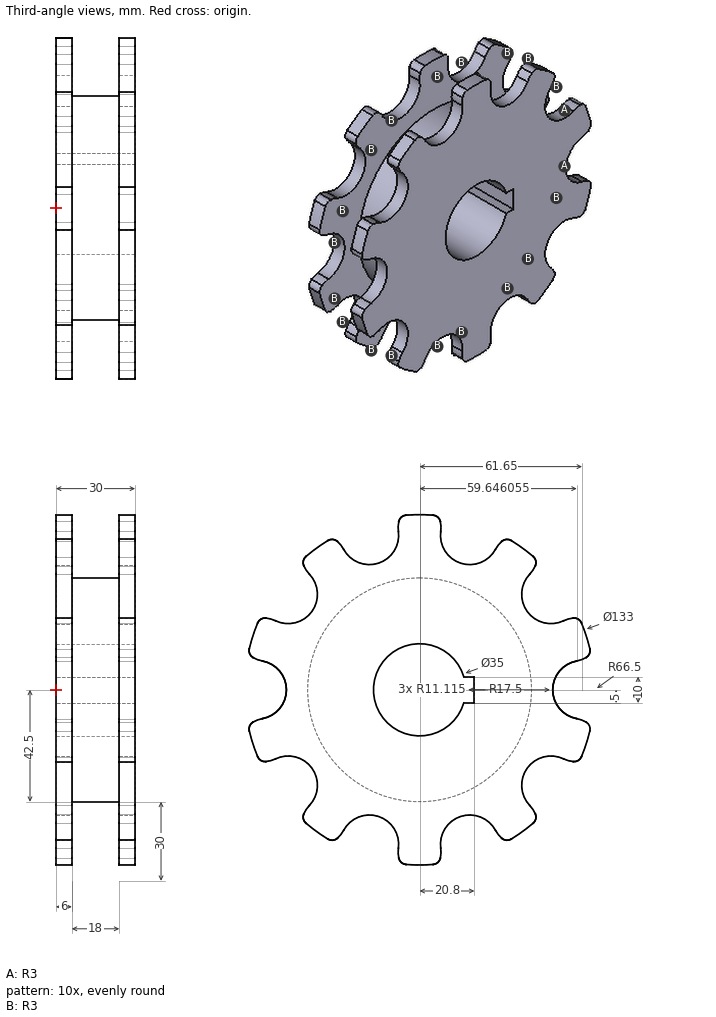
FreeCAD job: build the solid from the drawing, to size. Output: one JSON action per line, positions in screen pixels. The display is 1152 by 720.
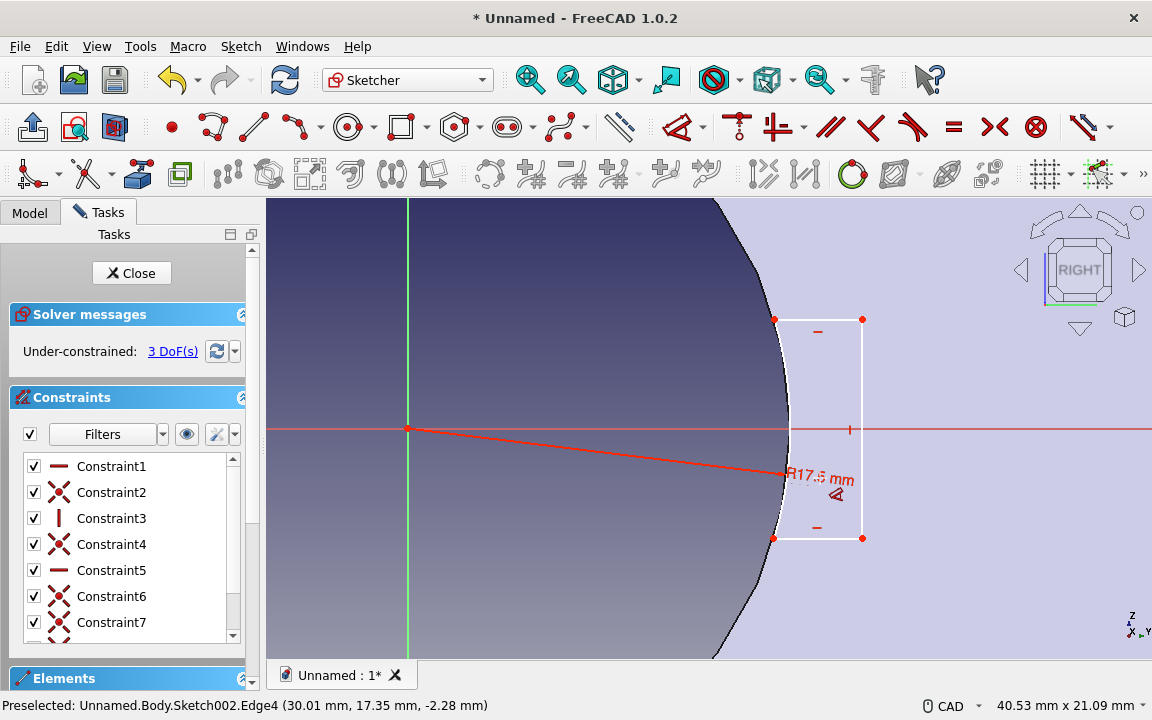
{"action": "left_click", "coordinate": [862, 473]}
{"action": "left_click", "coordinate": [896, 379]}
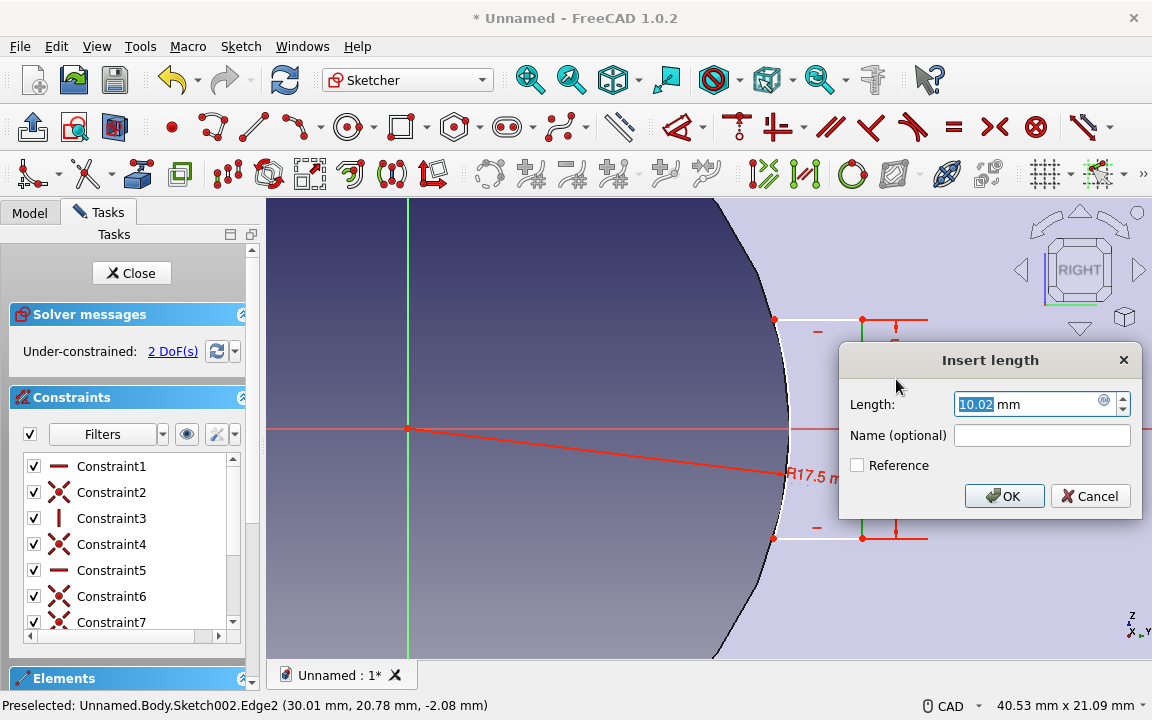
{"action": "type", "text": "10"}
{"action": "key", "text": "Return"}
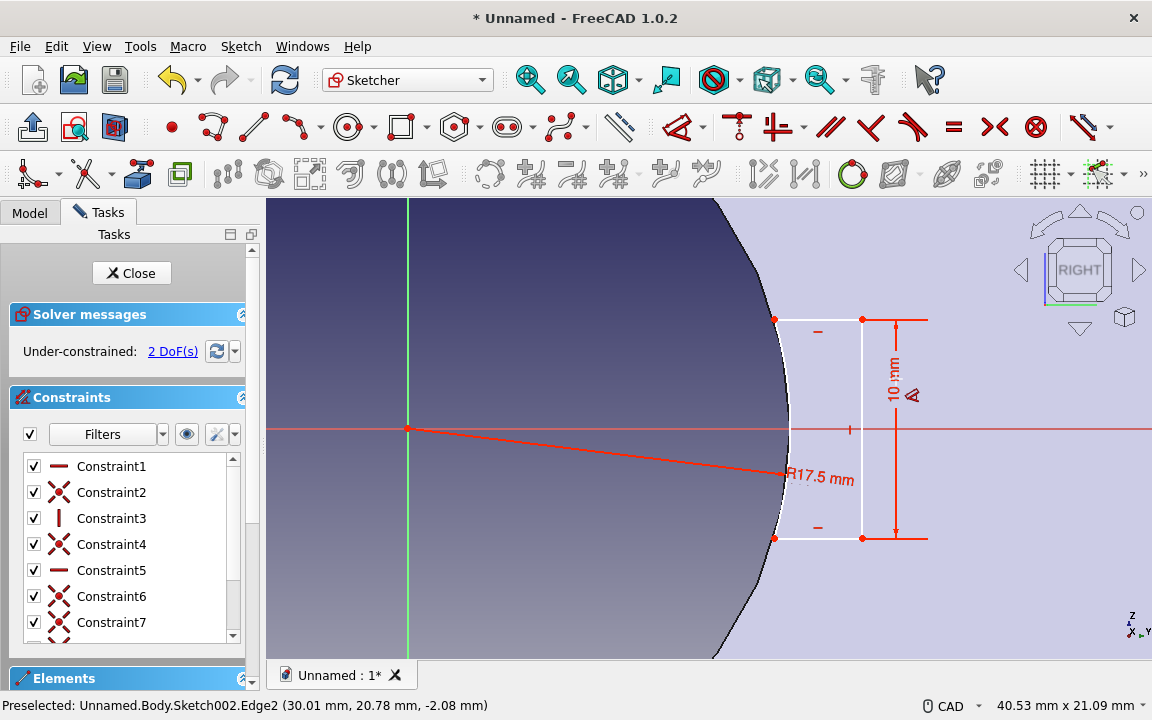
{"action": "left_click", "coordinate": [774, 539]}
{"action": "left_click", "coordinate": [374, 484]}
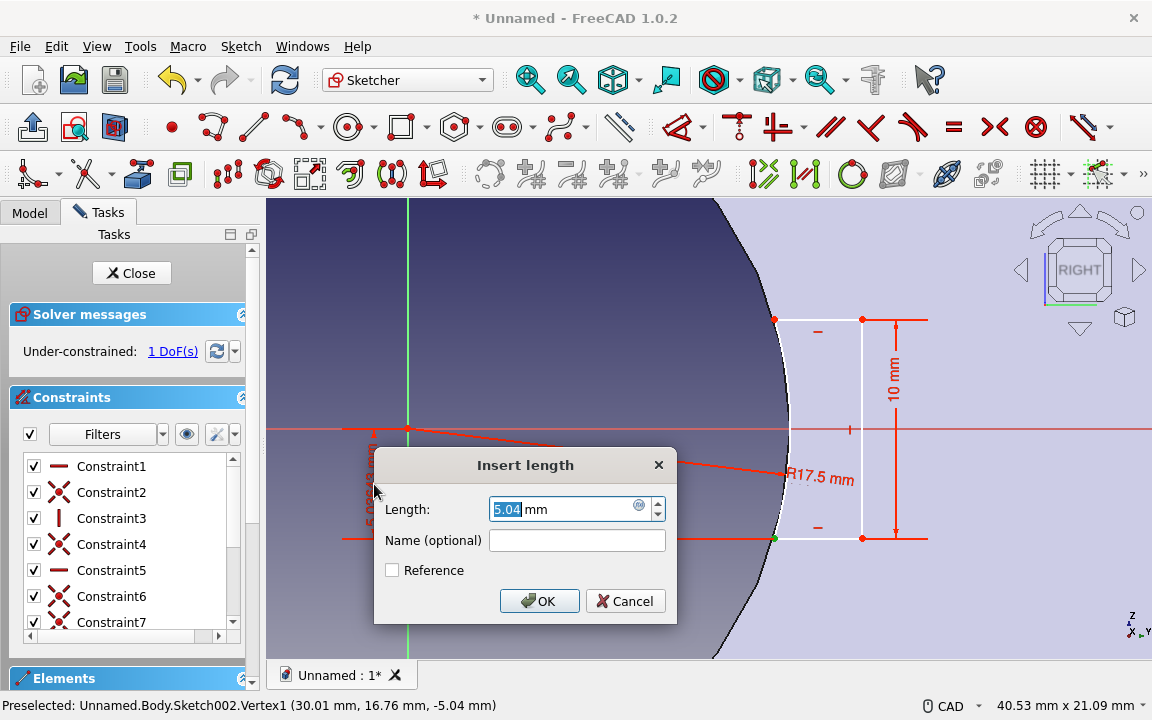
{"action": "type", "text": "5"}
{"action": "key", "text": "Return"}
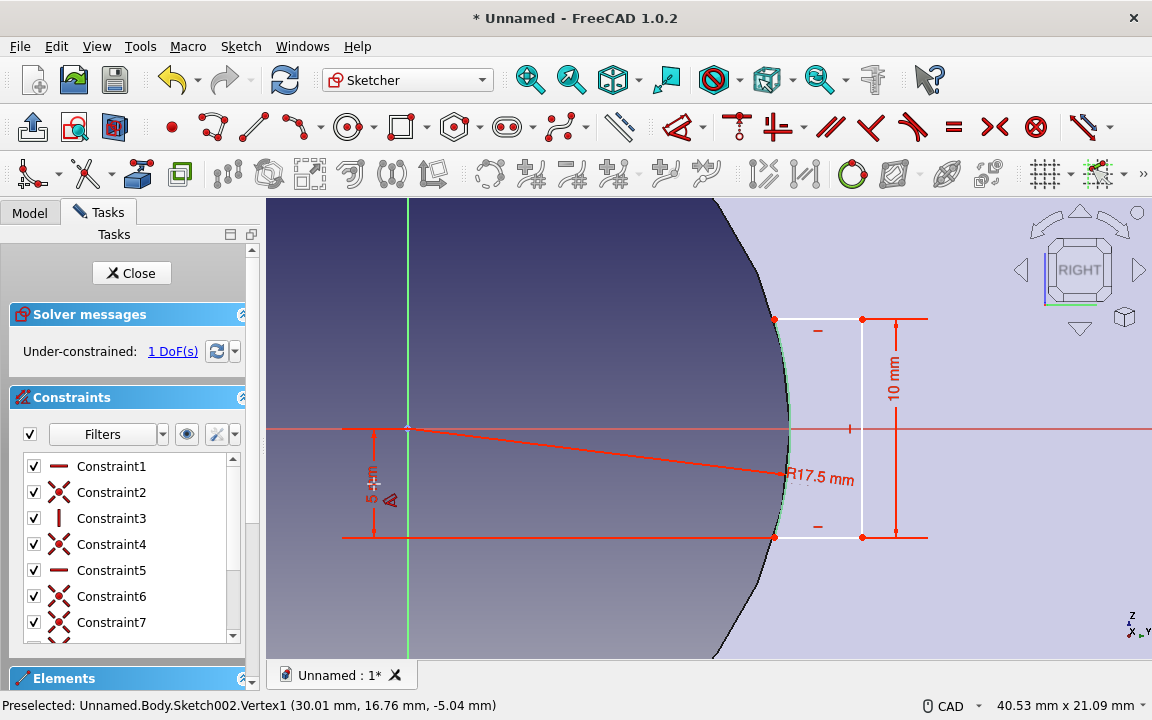
{"action": "left_click", "coordinate": [862, 538]}
{"action": "left_click", "coordinate": [635, 572]}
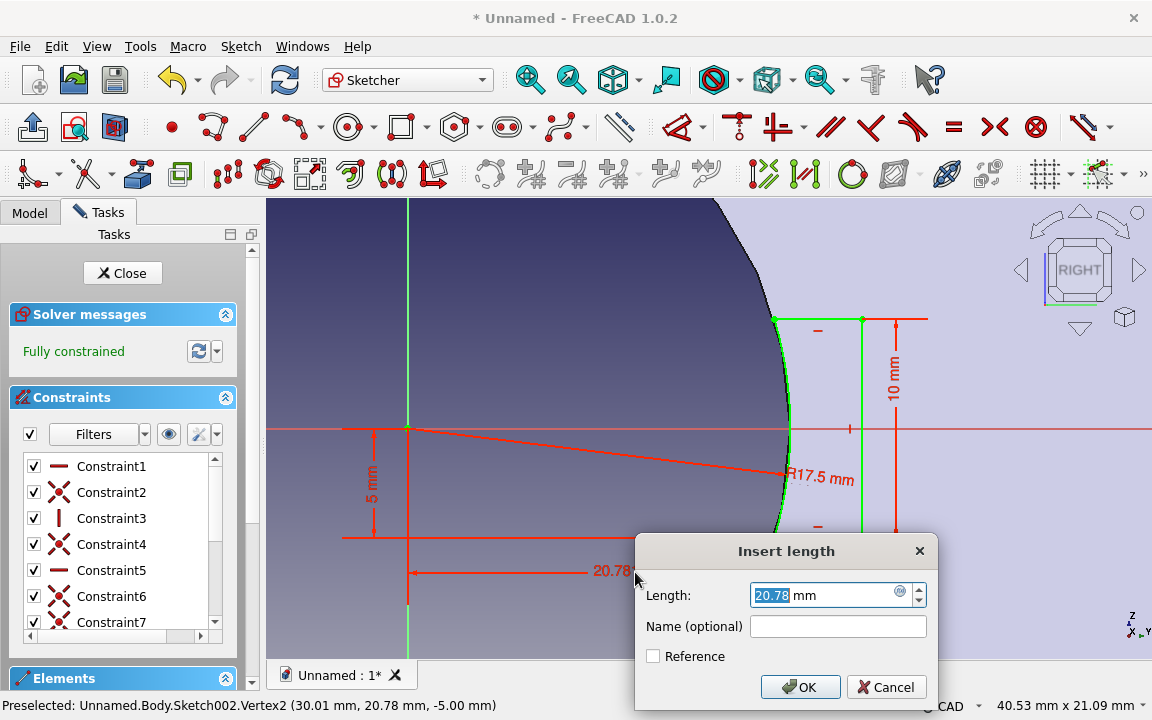
{"action": "type", "text": "20.8"}
{"action": "key", "text": "Return"}
{"action": "key", "text": "Escape"}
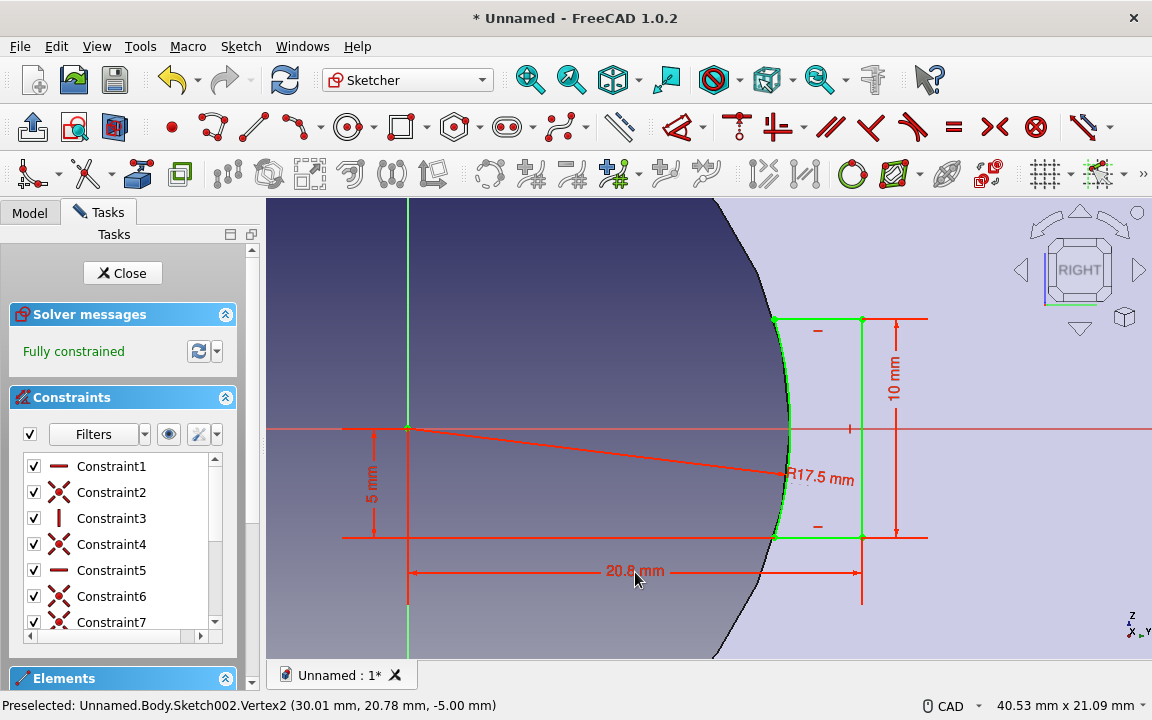
{"action": "left_click", "coordinate": [123, 273]}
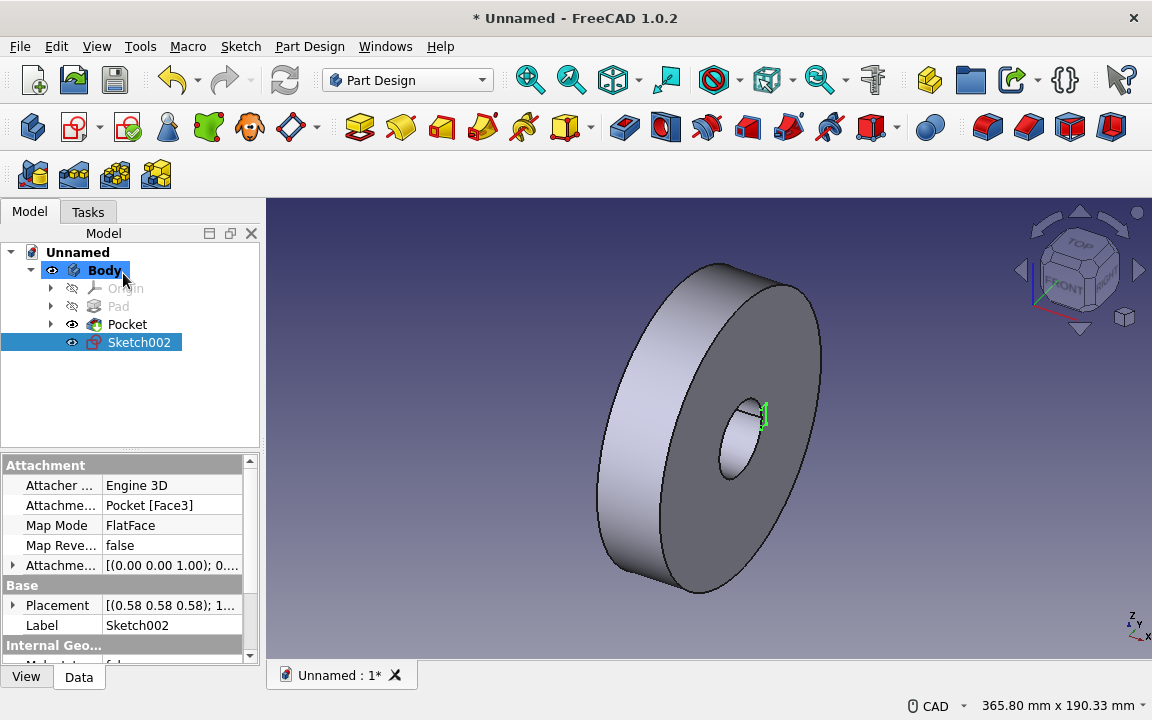
{"action": "left_click", "coordinate": [625, 128]}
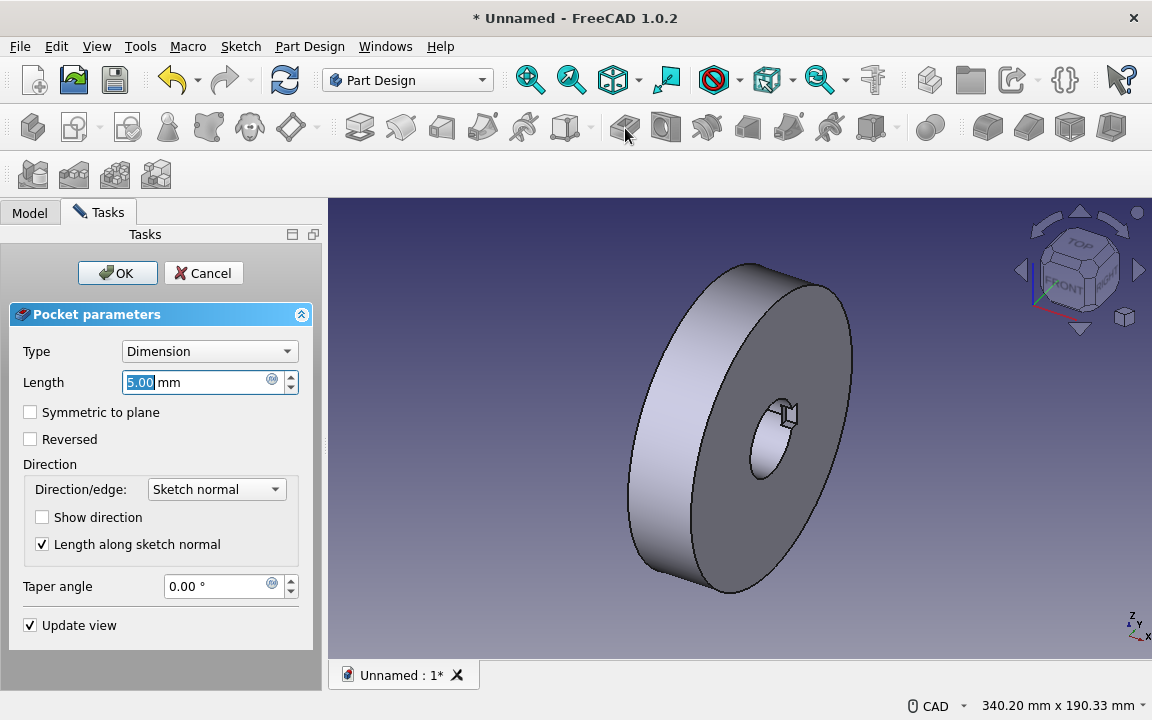
{"action": "left_click", "coordinate": [210, 352]}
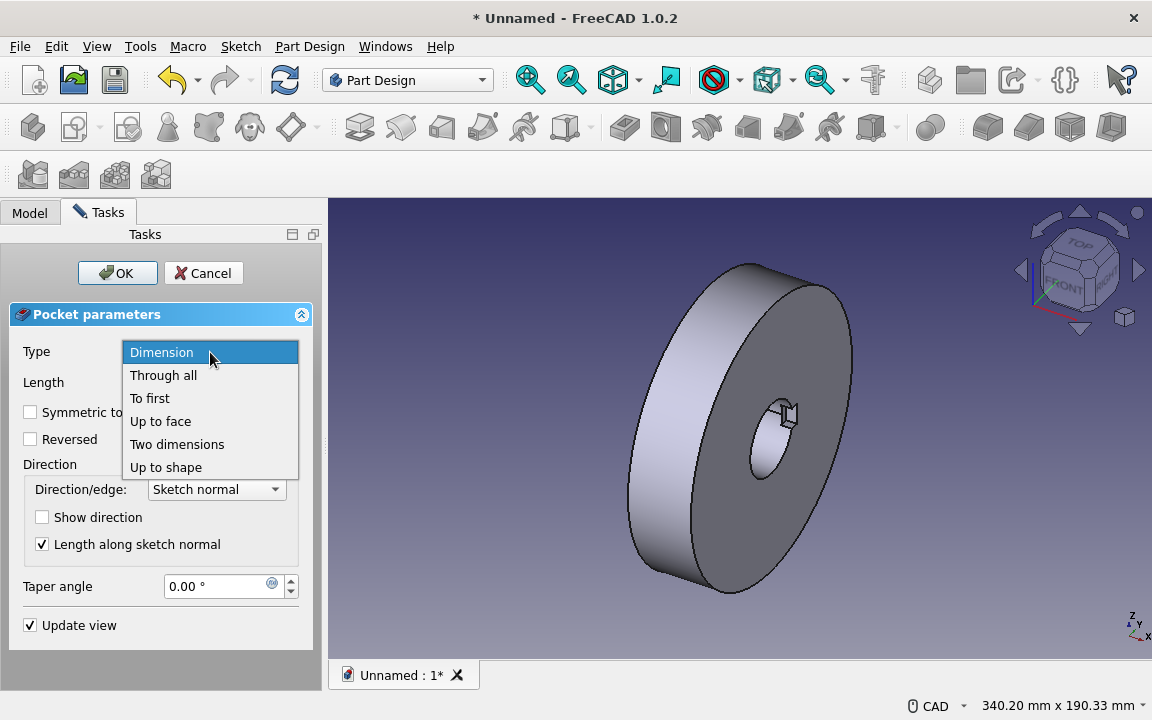
{"action": "left_click", "coordinate": [208, 376]}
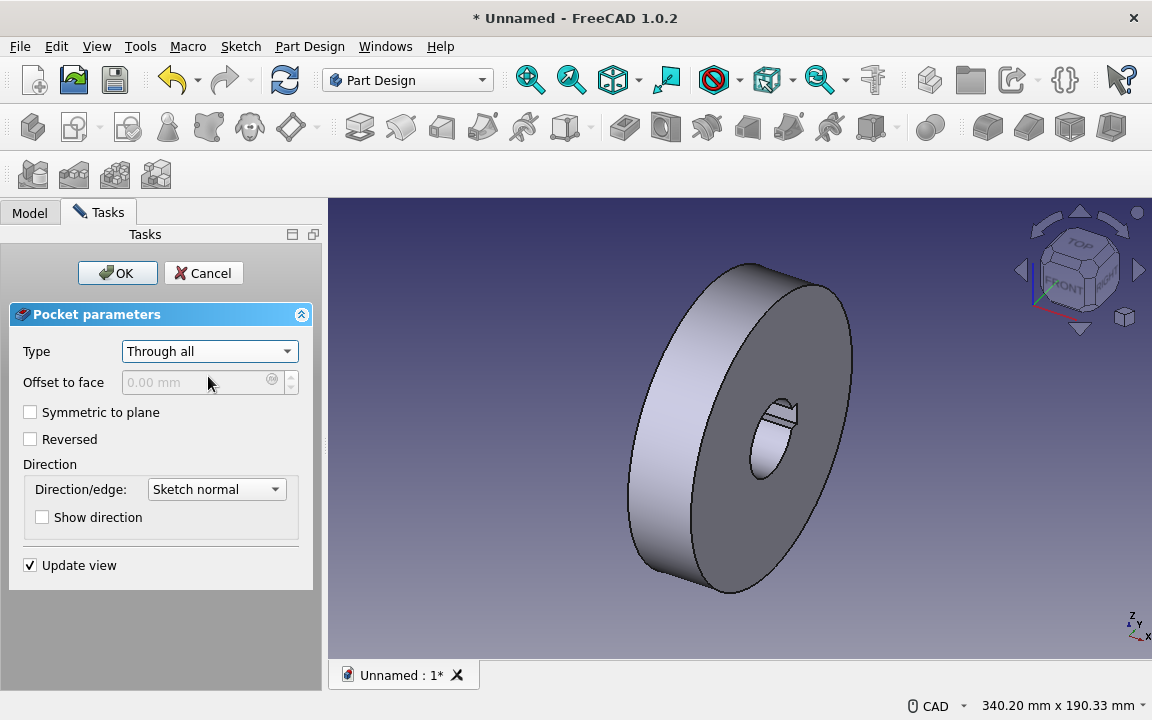
{"action": "left_click", "coordinate": [118, 273]}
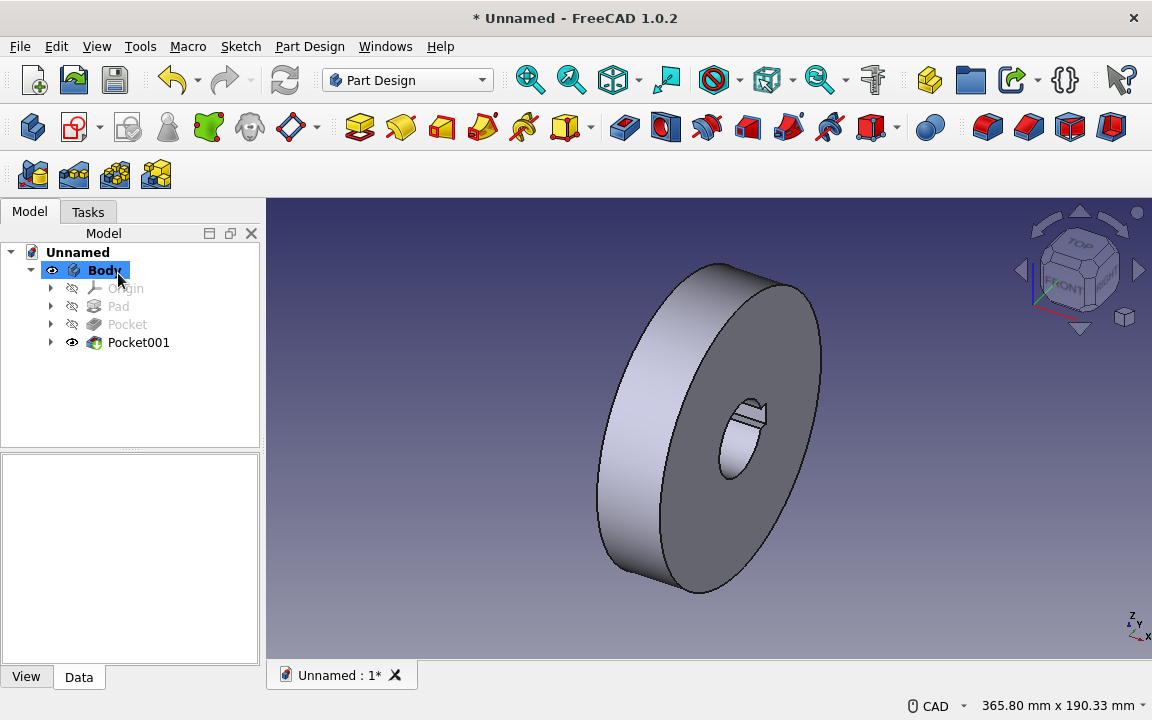
{"action": "left_click", "coordinate": [694, 446]}